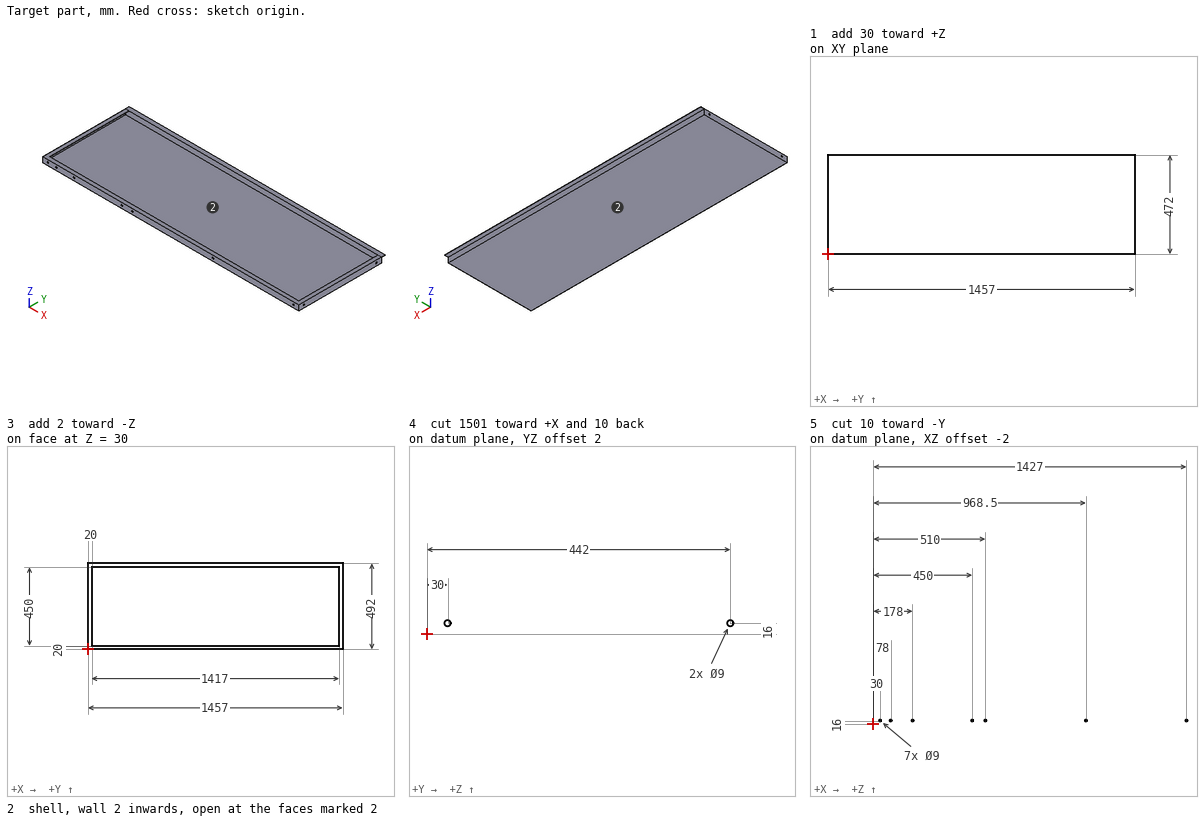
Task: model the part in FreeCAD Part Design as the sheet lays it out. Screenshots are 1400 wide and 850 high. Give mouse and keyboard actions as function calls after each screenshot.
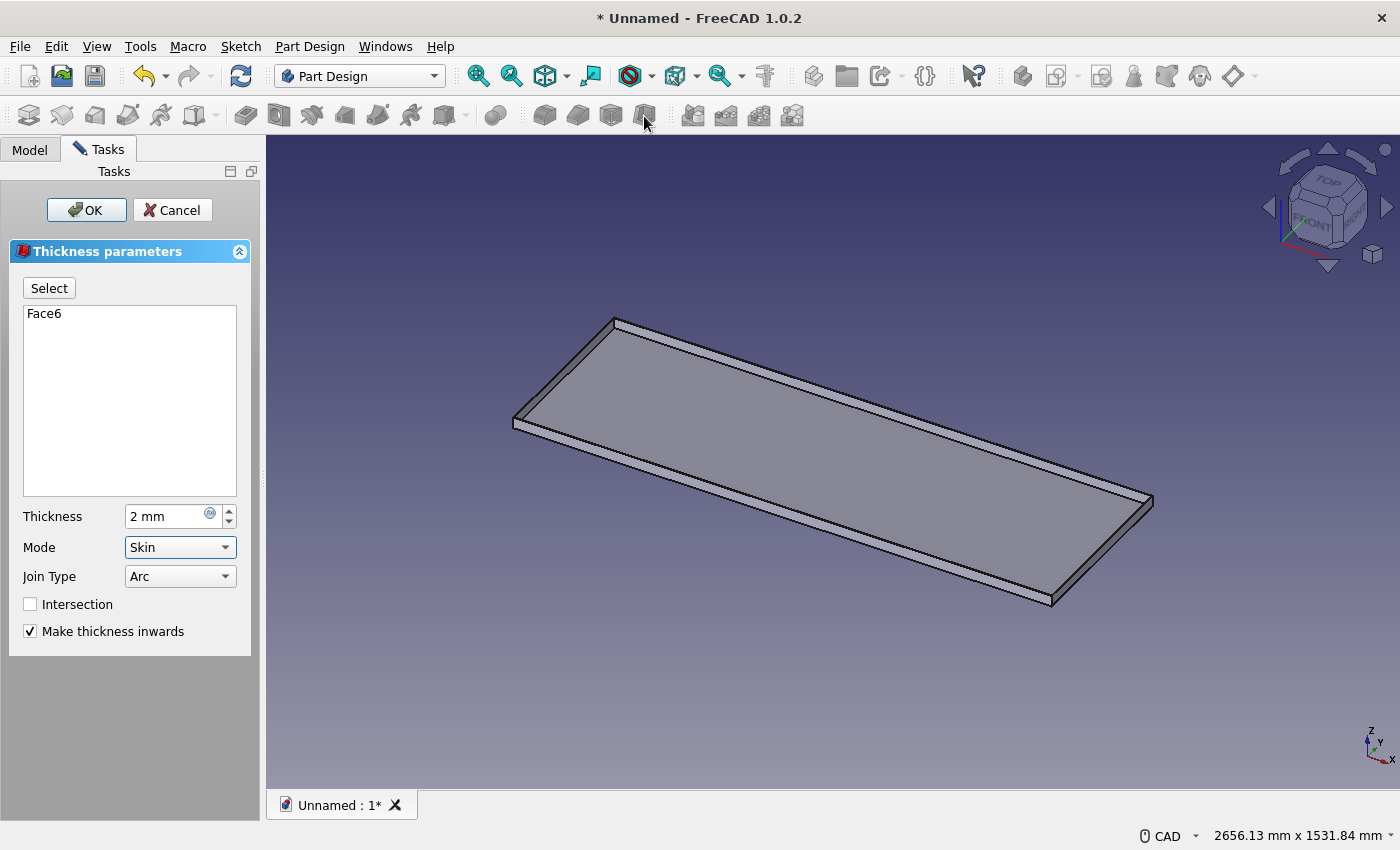
click(181, 576)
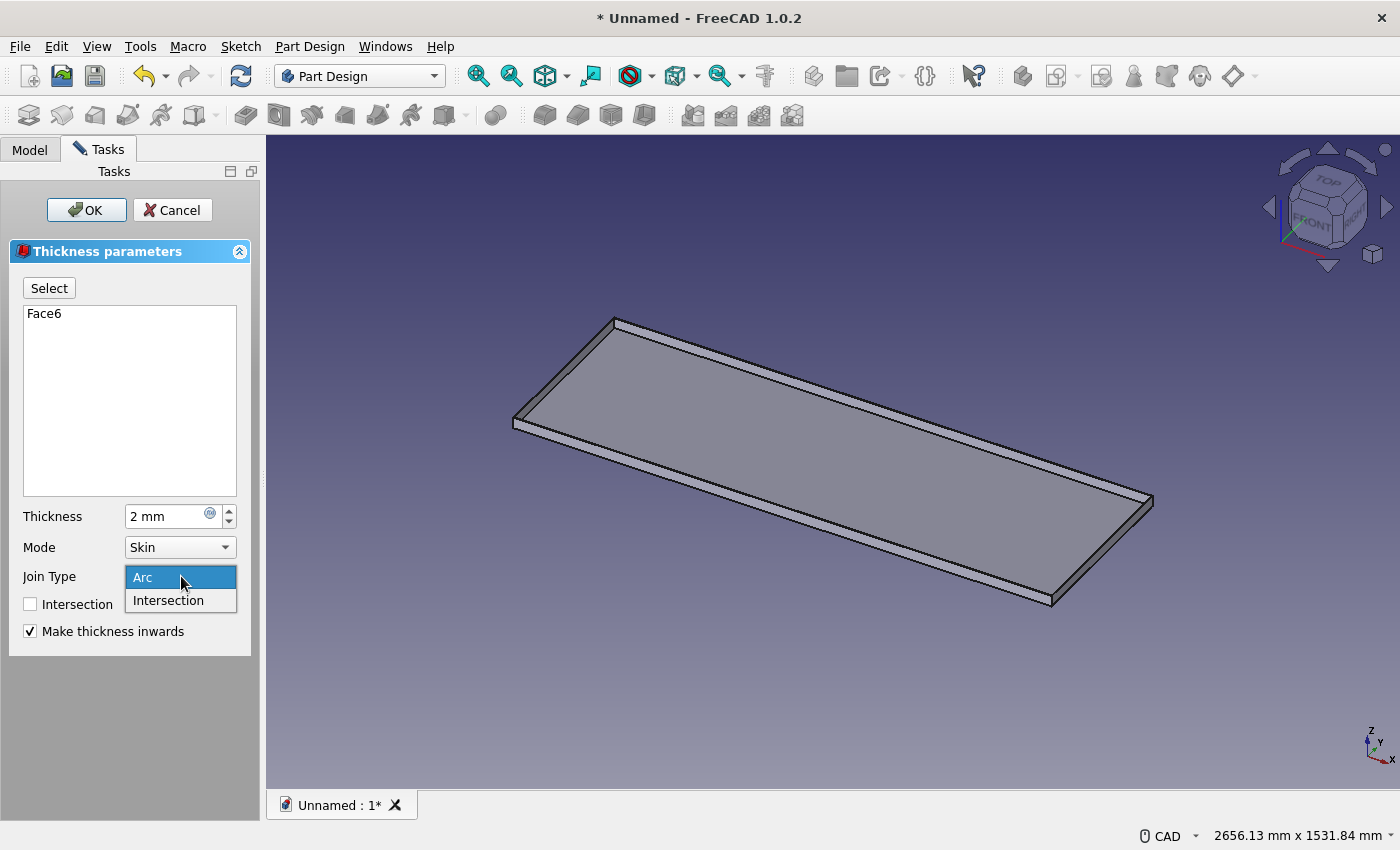
click(179, 600)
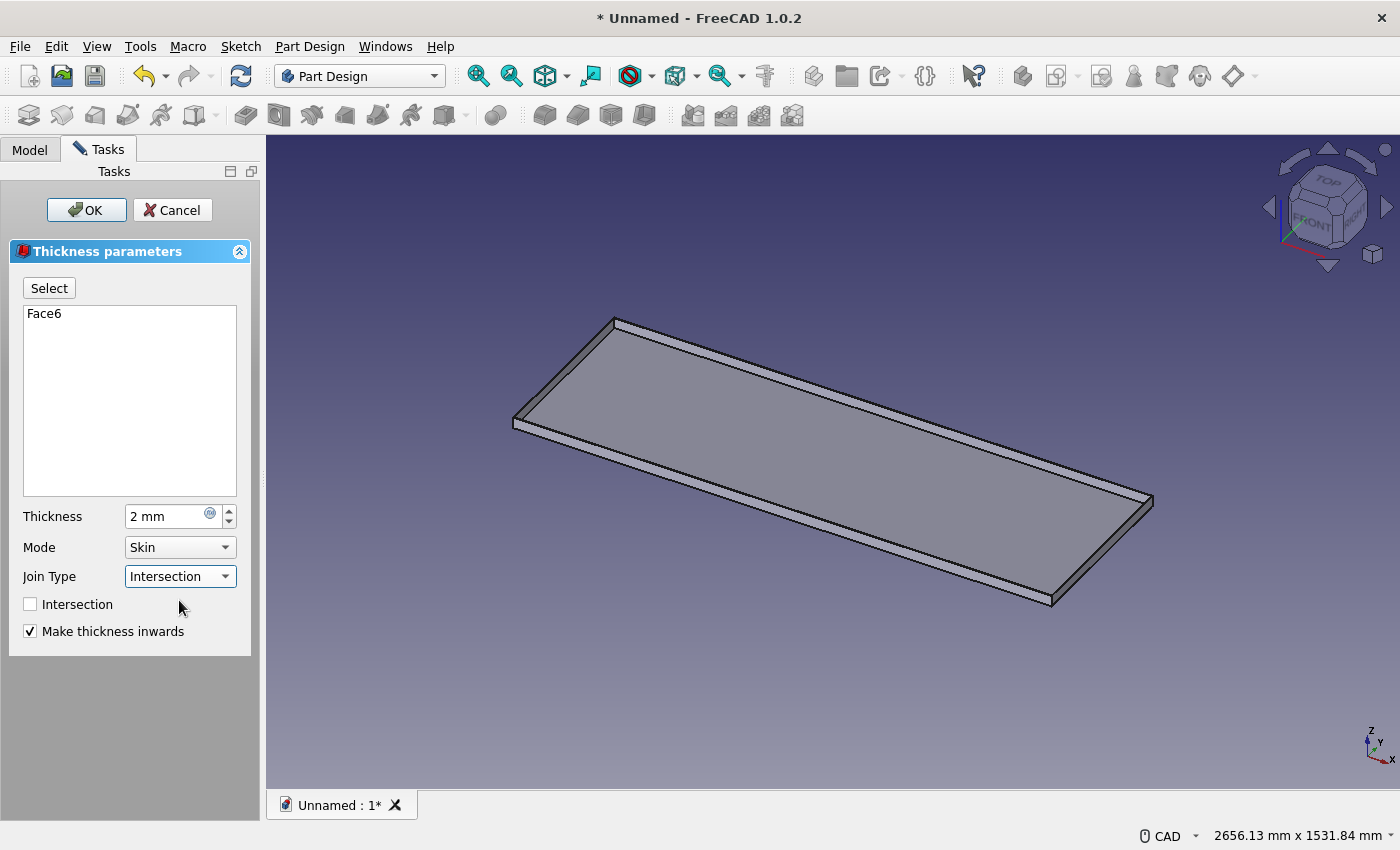
click(87, 210)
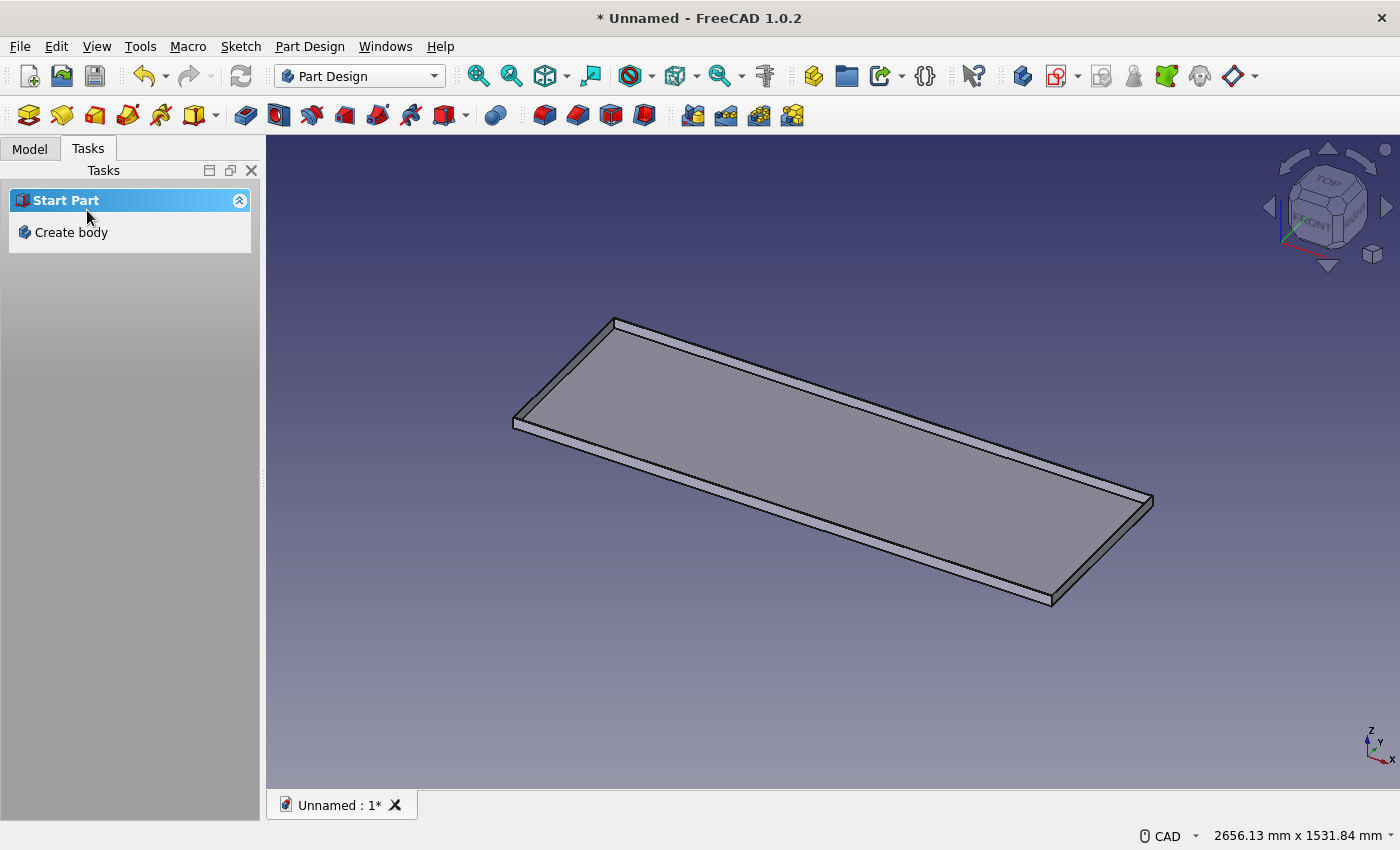
scroll(1085, 561, up, 15)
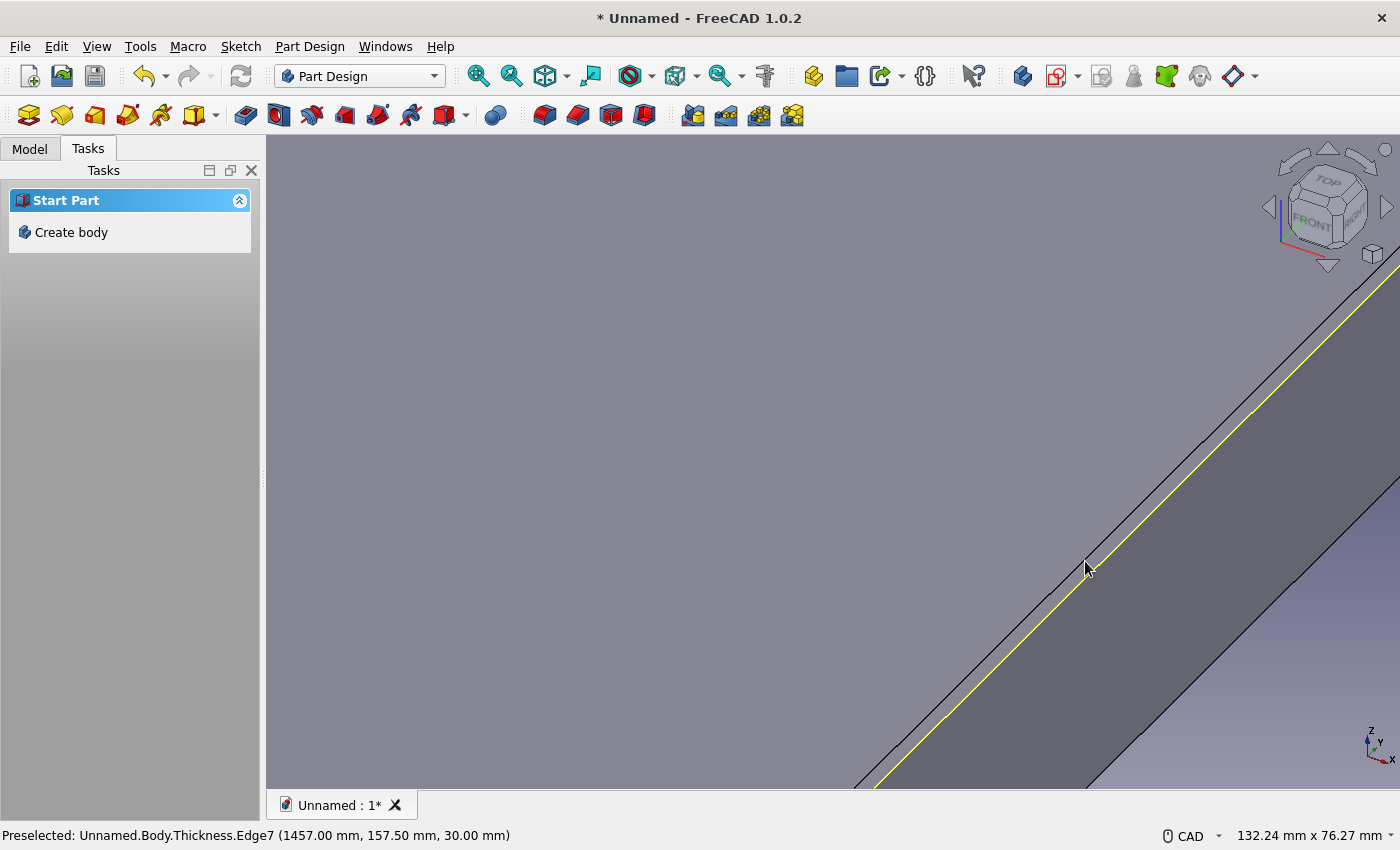
scroll(1080, 576, up, 4)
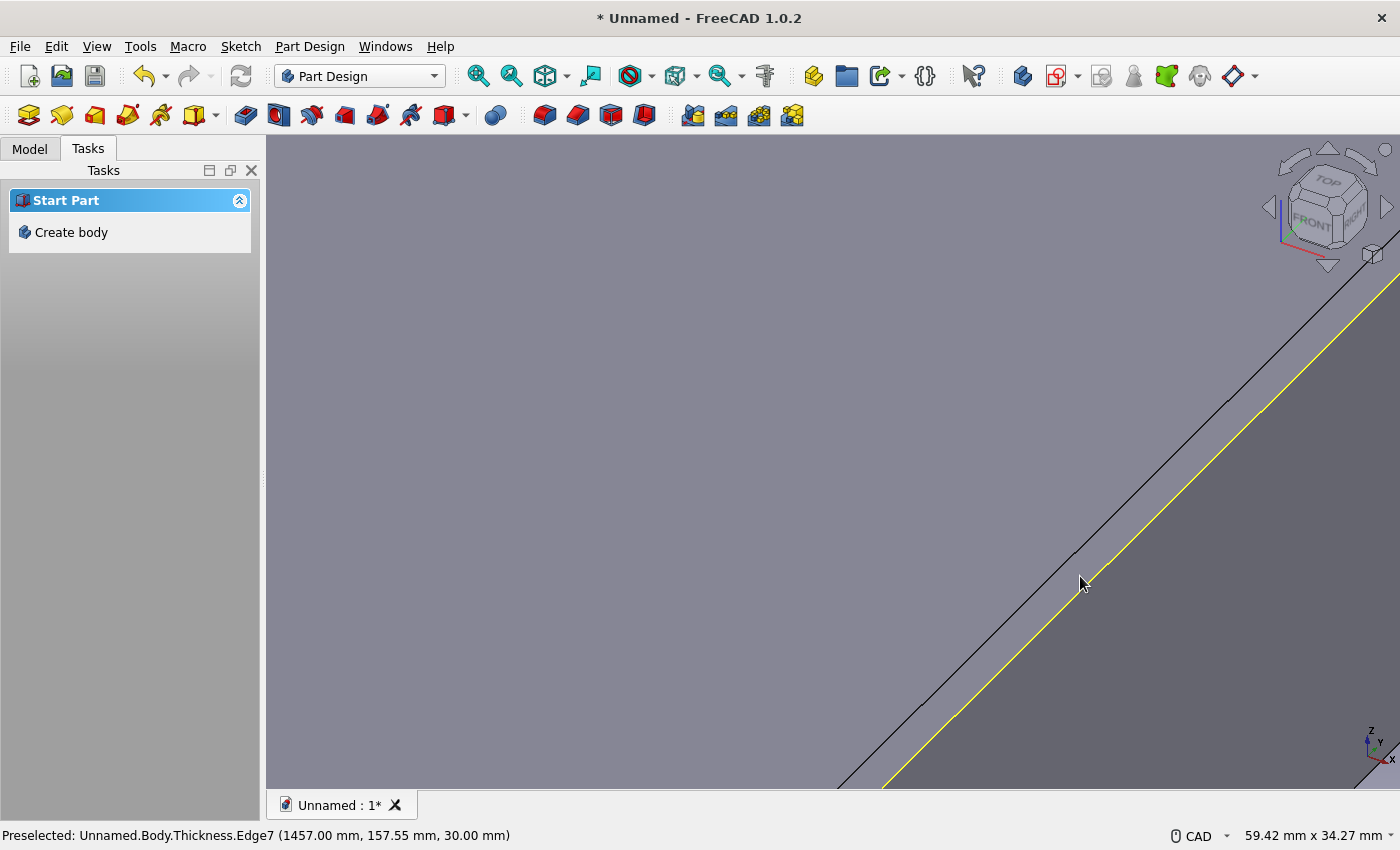
click(1080, 576)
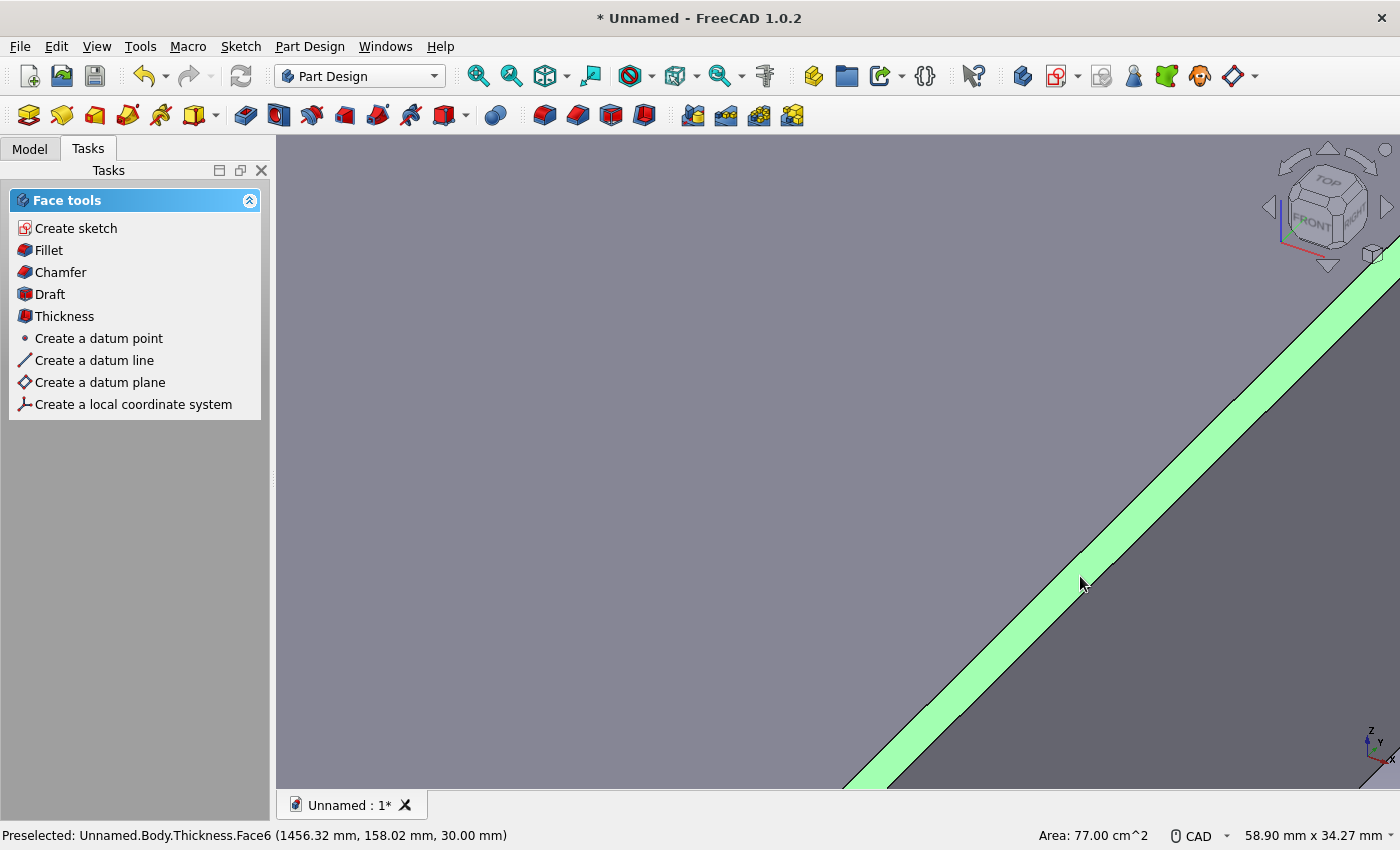
click(1056, 76)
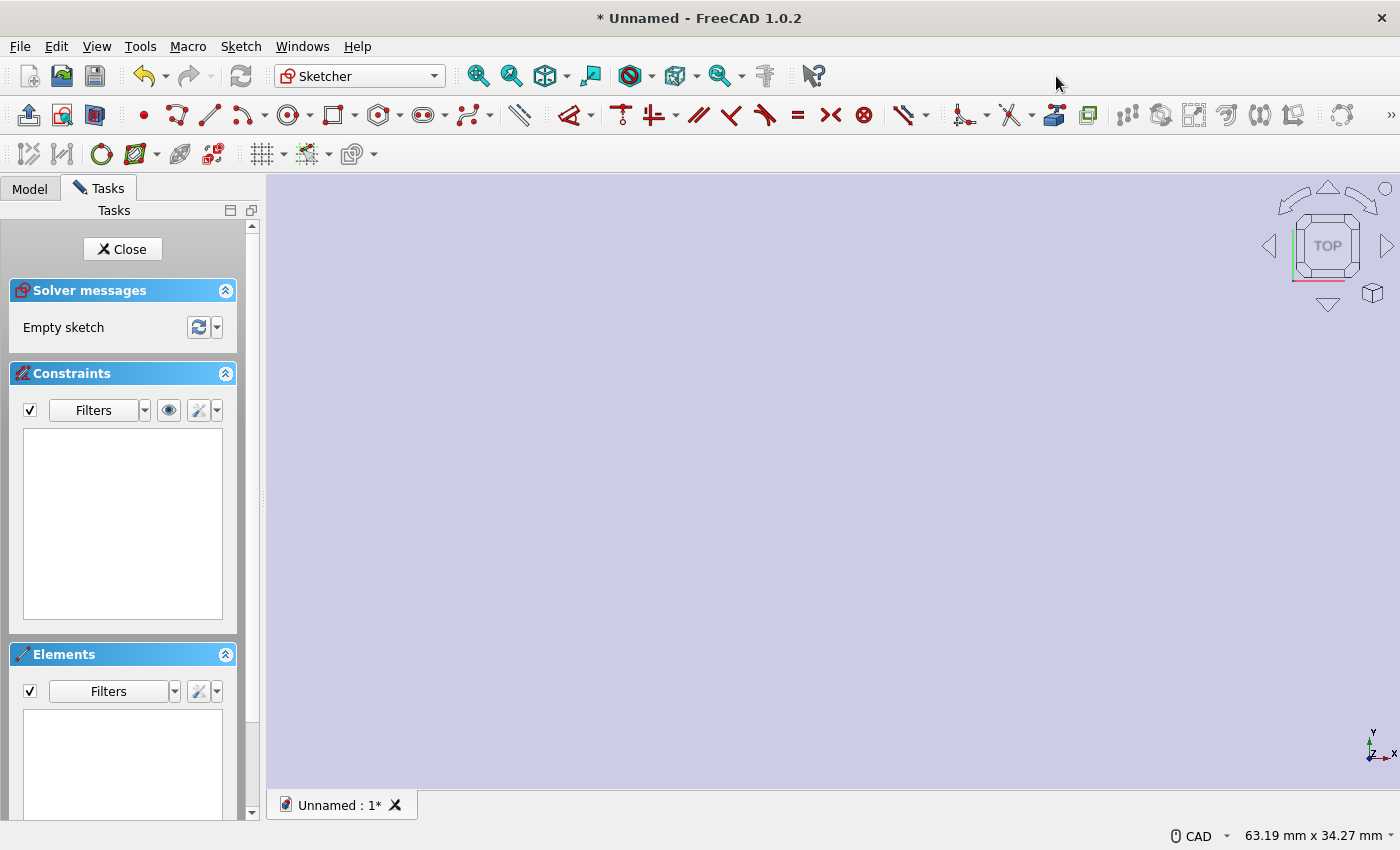
scroll(1113, 379, down, 17)